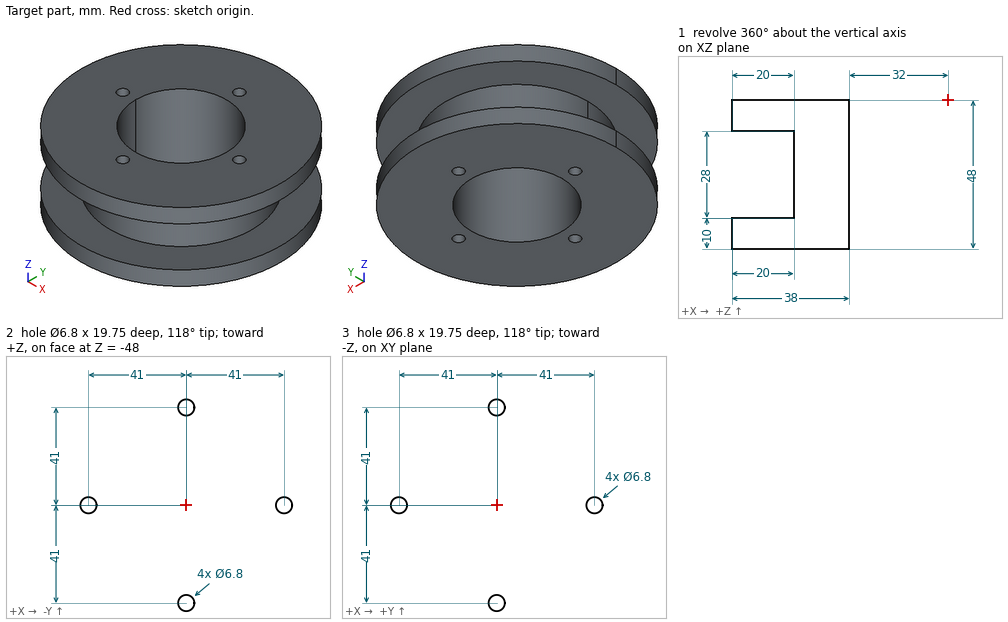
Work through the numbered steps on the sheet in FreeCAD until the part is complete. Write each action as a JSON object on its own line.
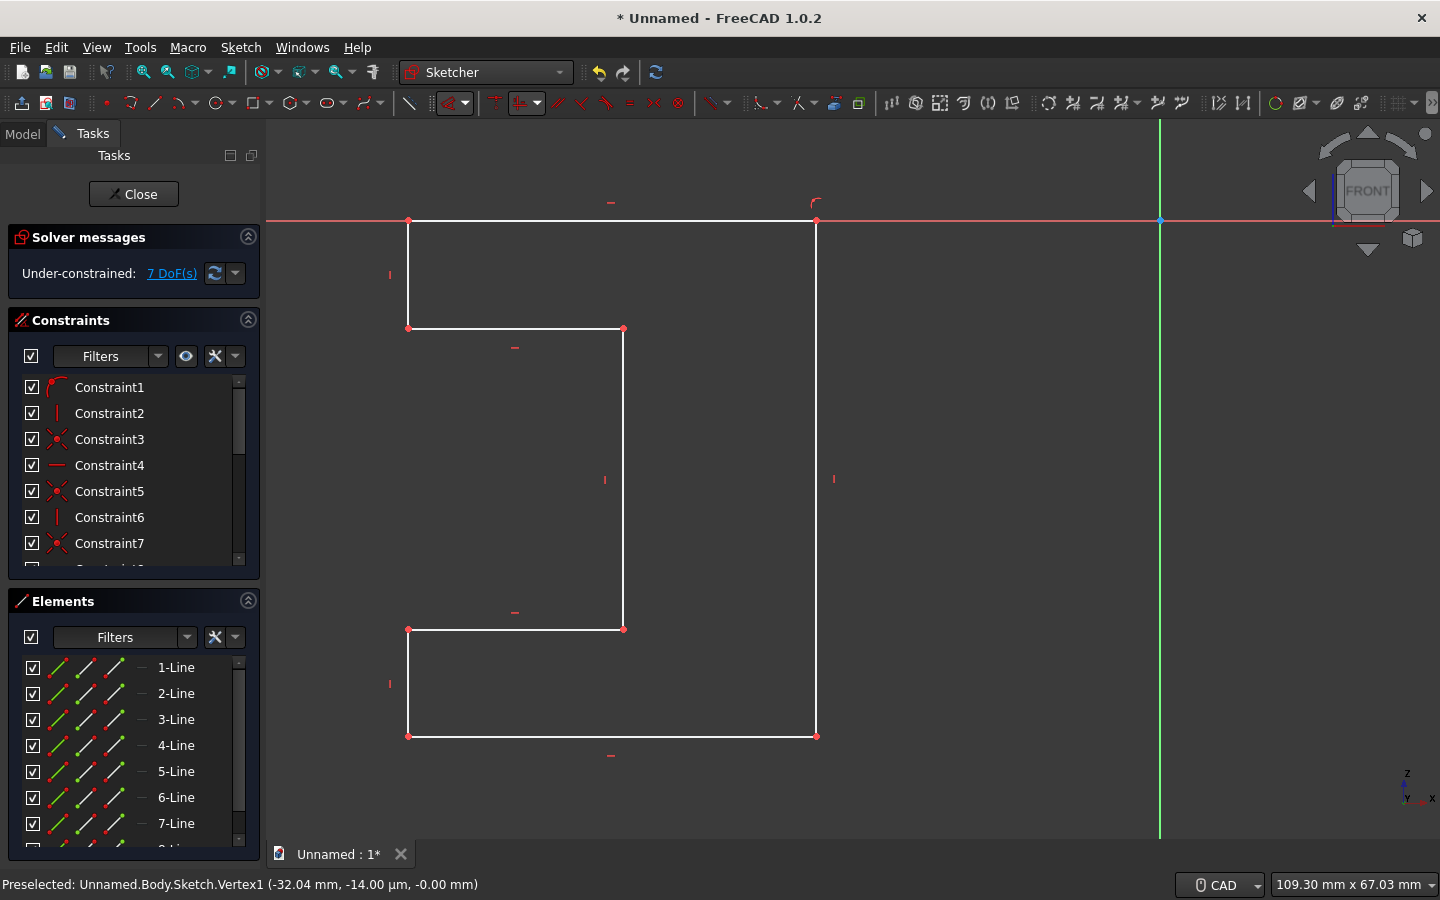
{"action": "left_click", "coordinate": [448, 104]}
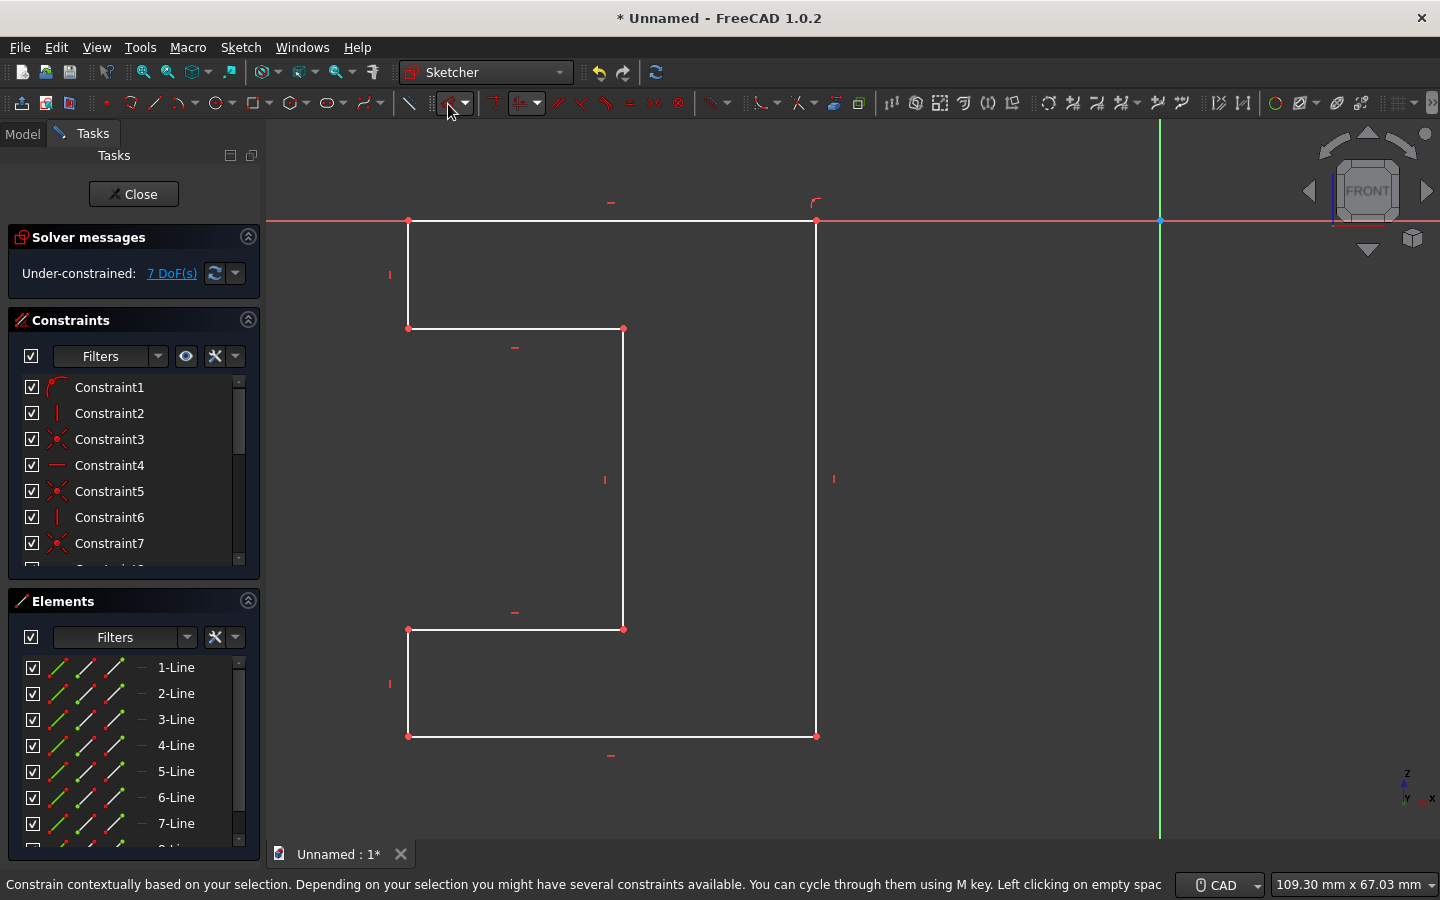
{"action": "left_click", "coordinate": [816, 376]}
{"action": "left_click", "coordinate": [850, 479]}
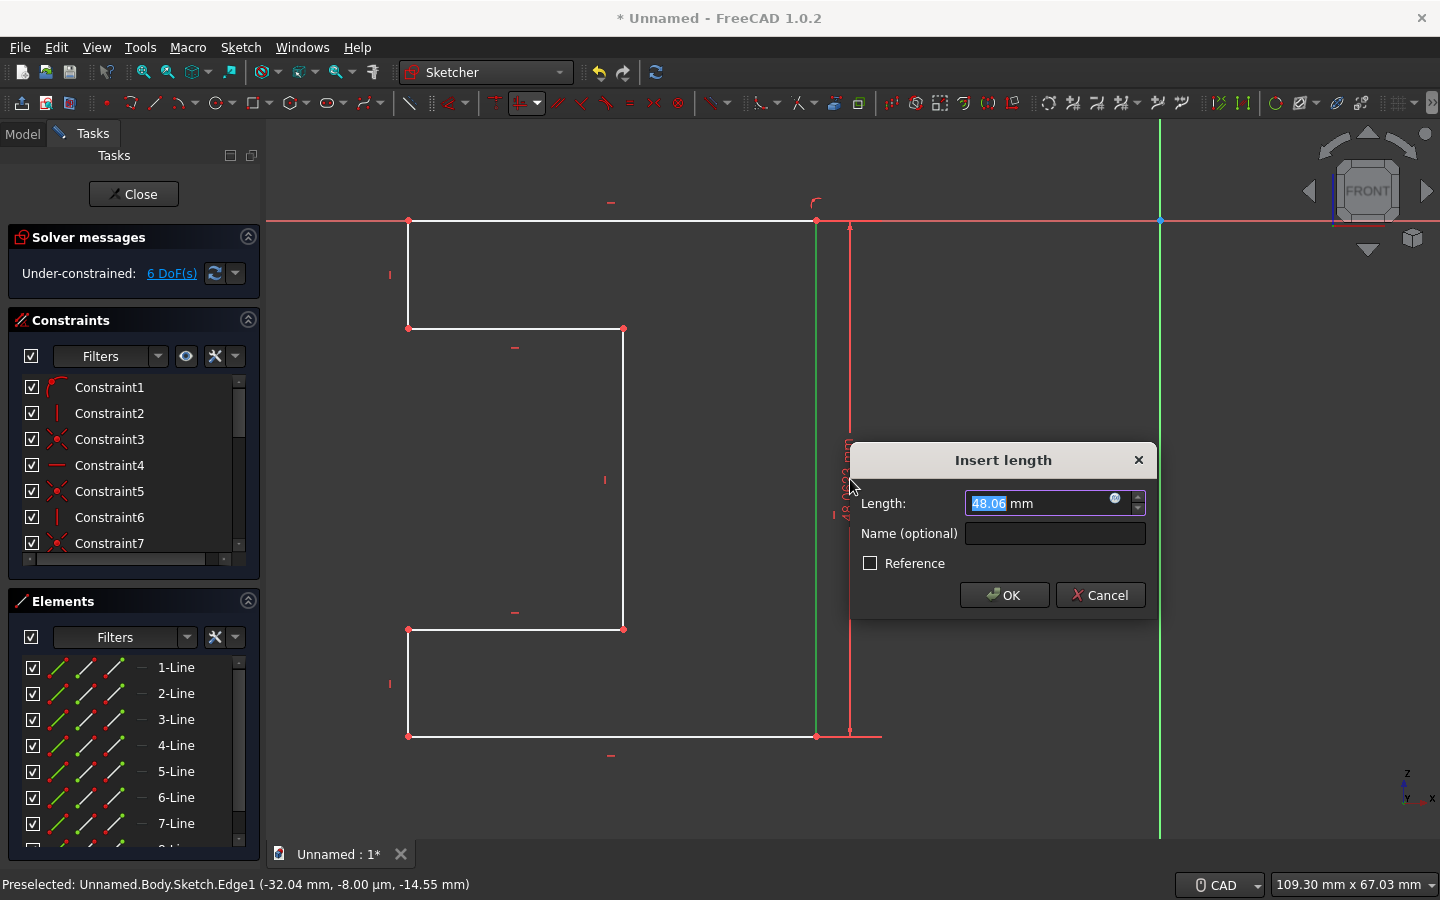
{"action": "type", "text": "48"}
{"action": "key", "text": "Return"}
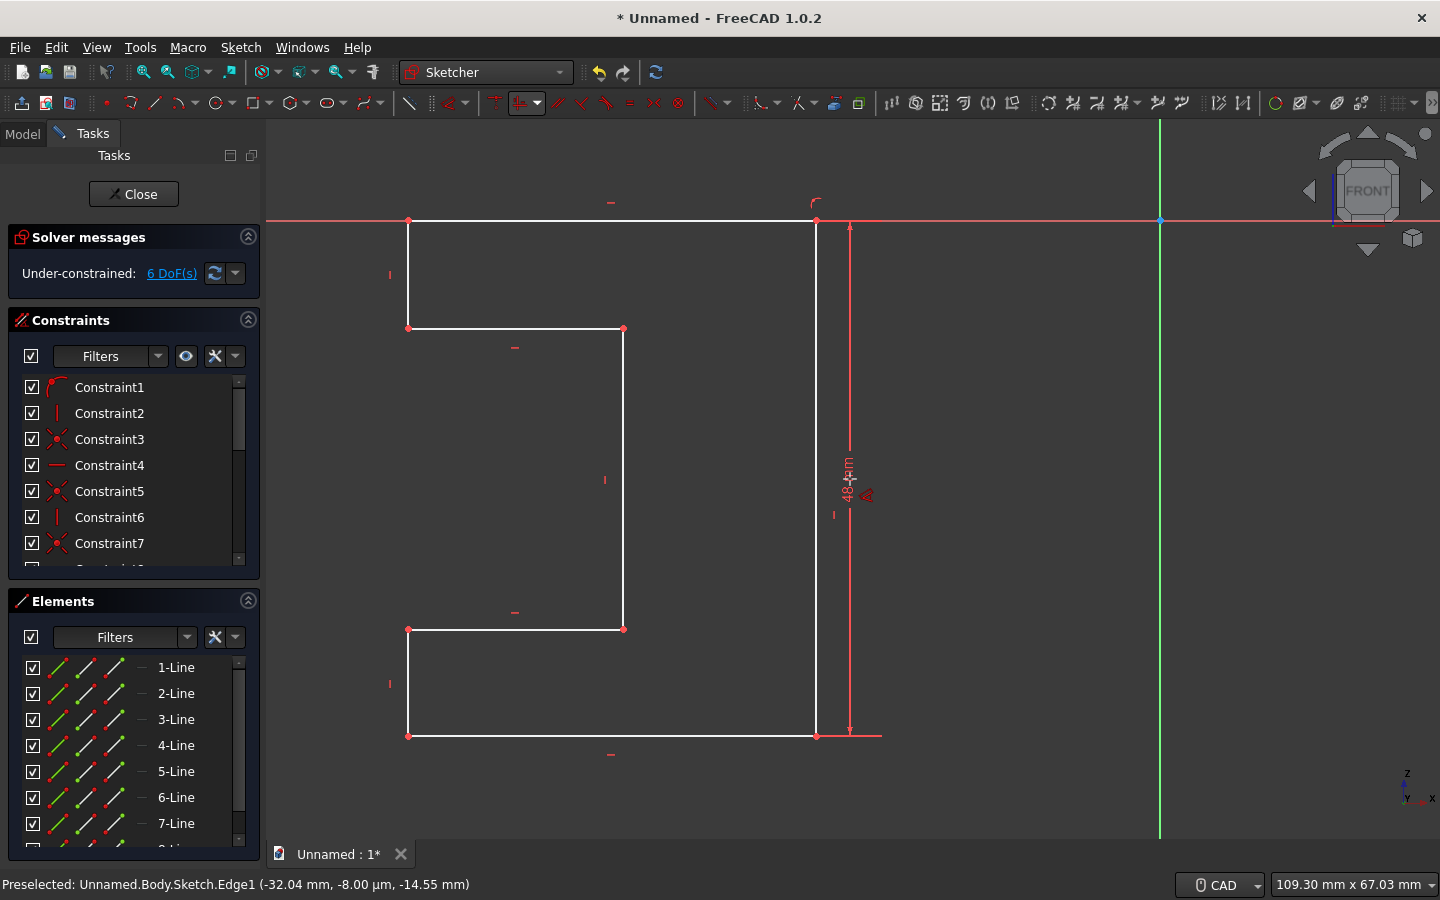
{"action": "left_click", "coordinate": [694, 736]}
{"action": "left_click", "coordinate": [612, 770]}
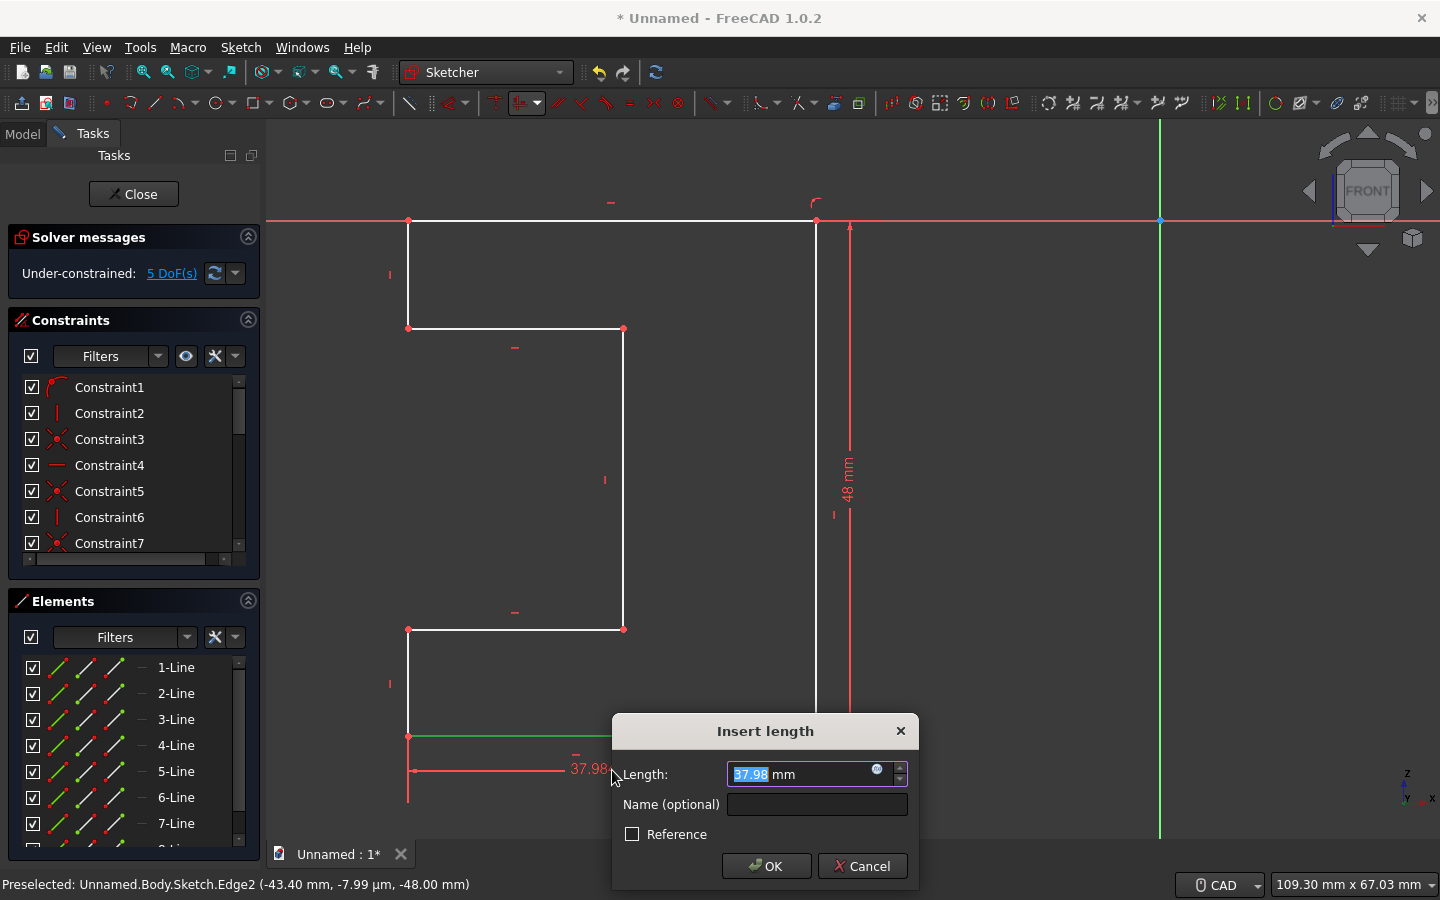
{"action": "type", "text": "38"}
{"action": "key", "text": "Return"}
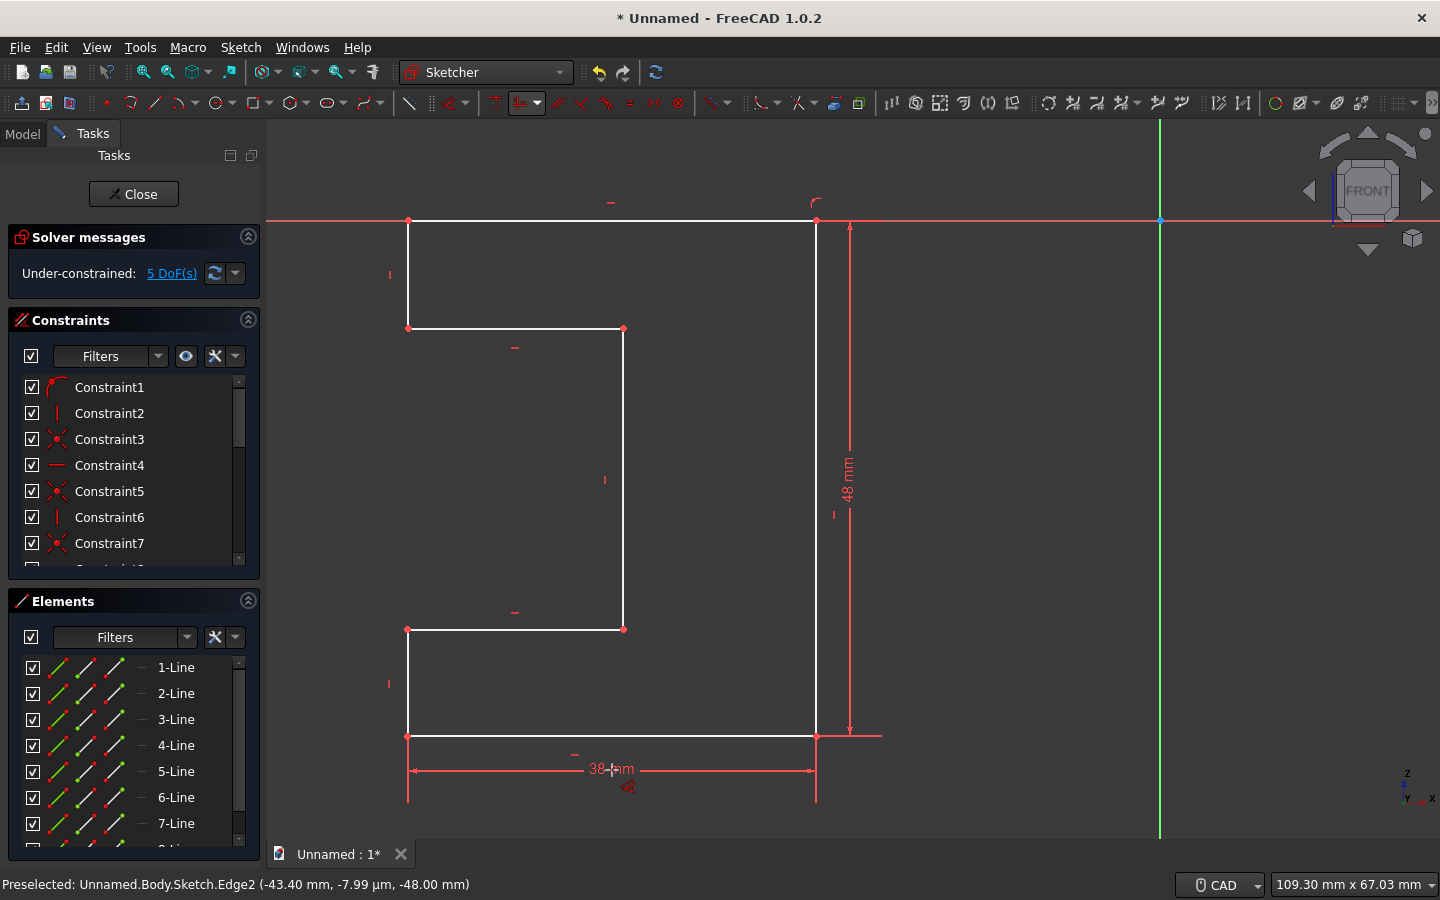
{"action": "left_click", "coordinate": [408, 704]}
{"action": "left_click", "coordinate": [374, 683]}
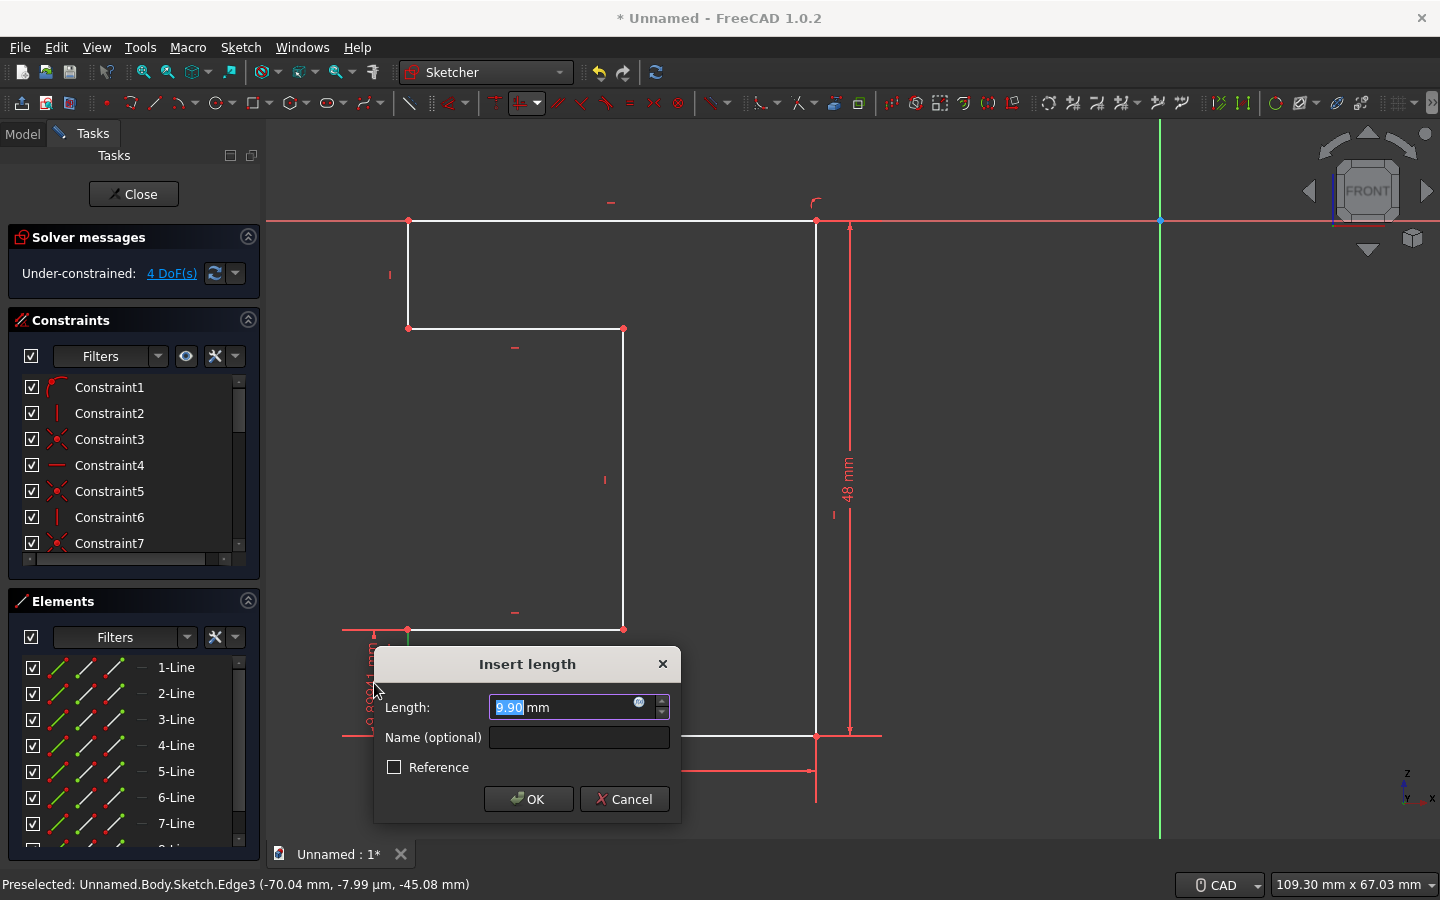
{"action": "type", "text": "10"}
{"action": "key", "text": "Return"}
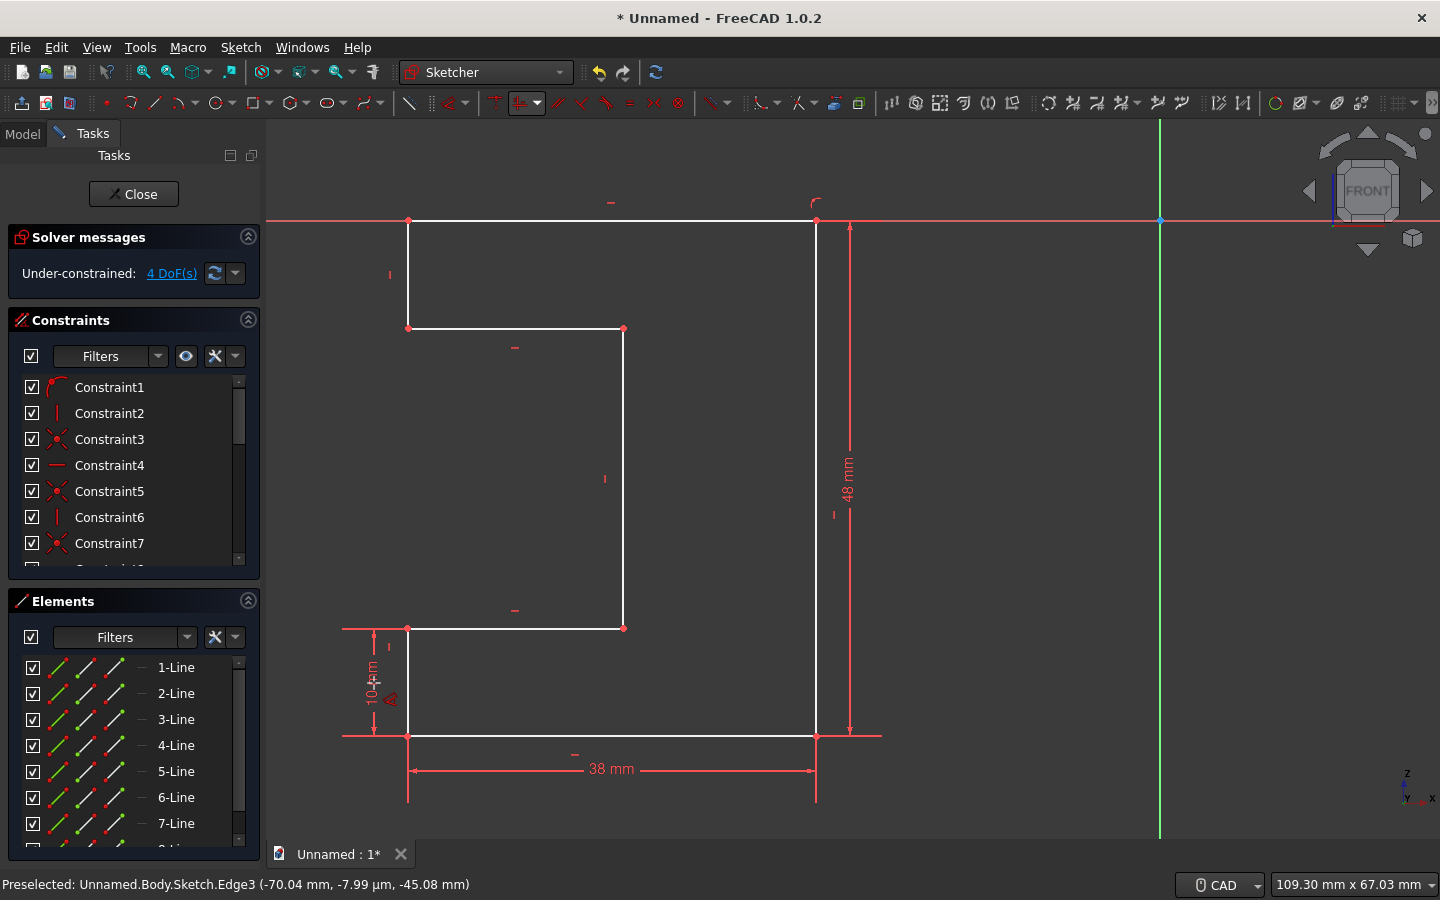
{"action": "left_click", "coordinate": [472, 629]}
{"action": "left_click", "coordinate": [515, 663]}